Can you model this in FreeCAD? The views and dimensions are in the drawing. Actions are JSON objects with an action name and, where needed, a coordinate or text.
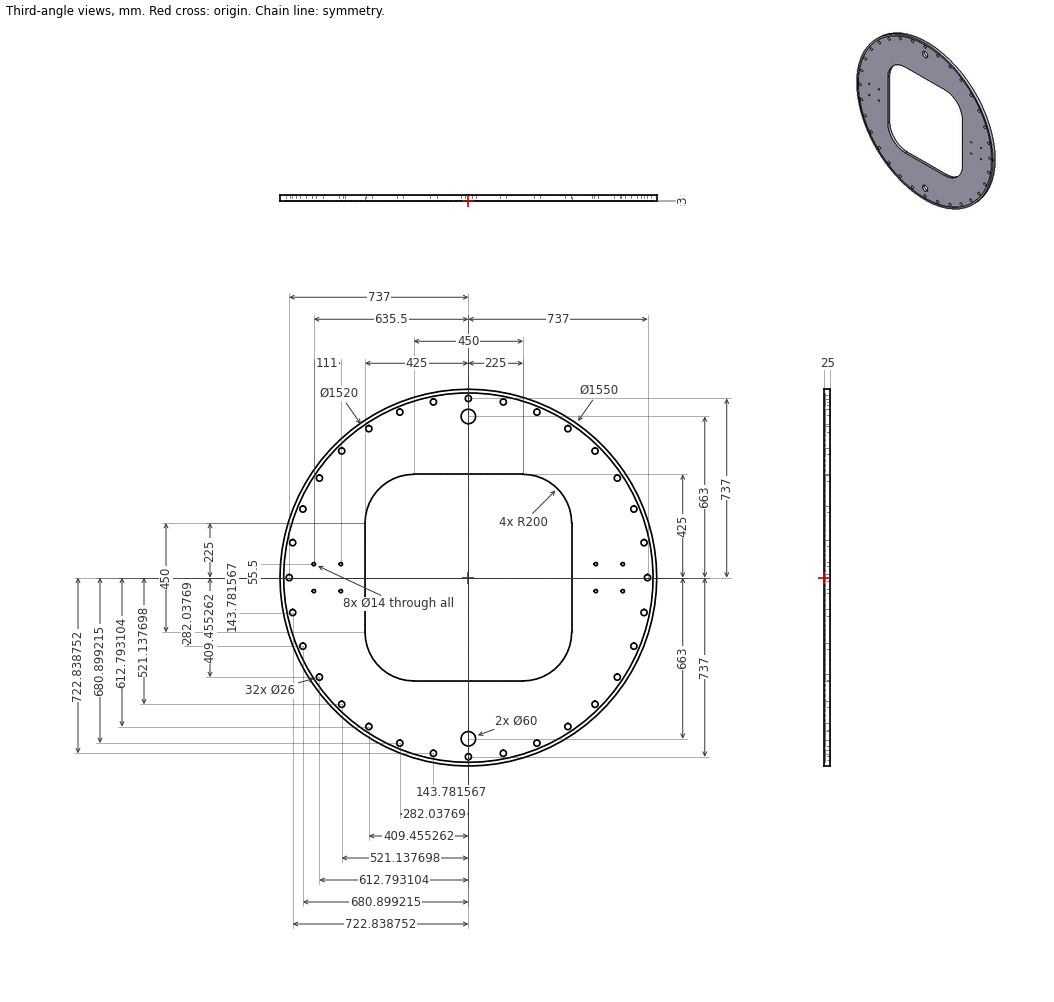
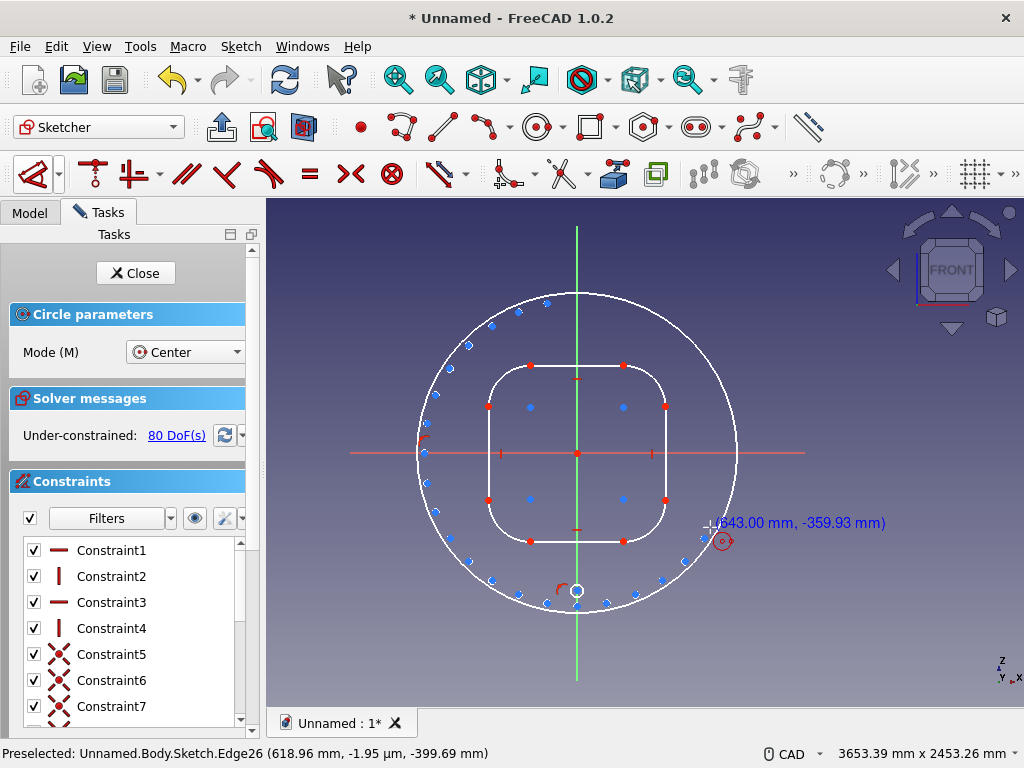
{"action": "scroll", "coordinate": [718, 512], "scroll_direction": "up", "scroll_amount": 4}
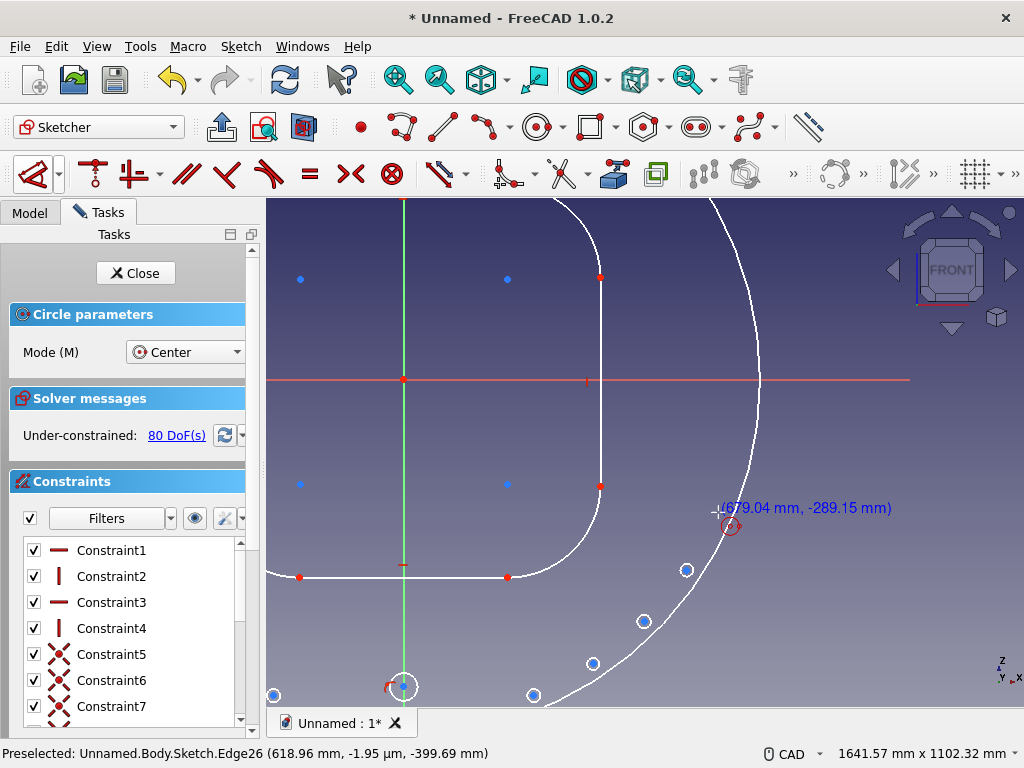
{"action": "left_click", "coordinate": [718, 510]}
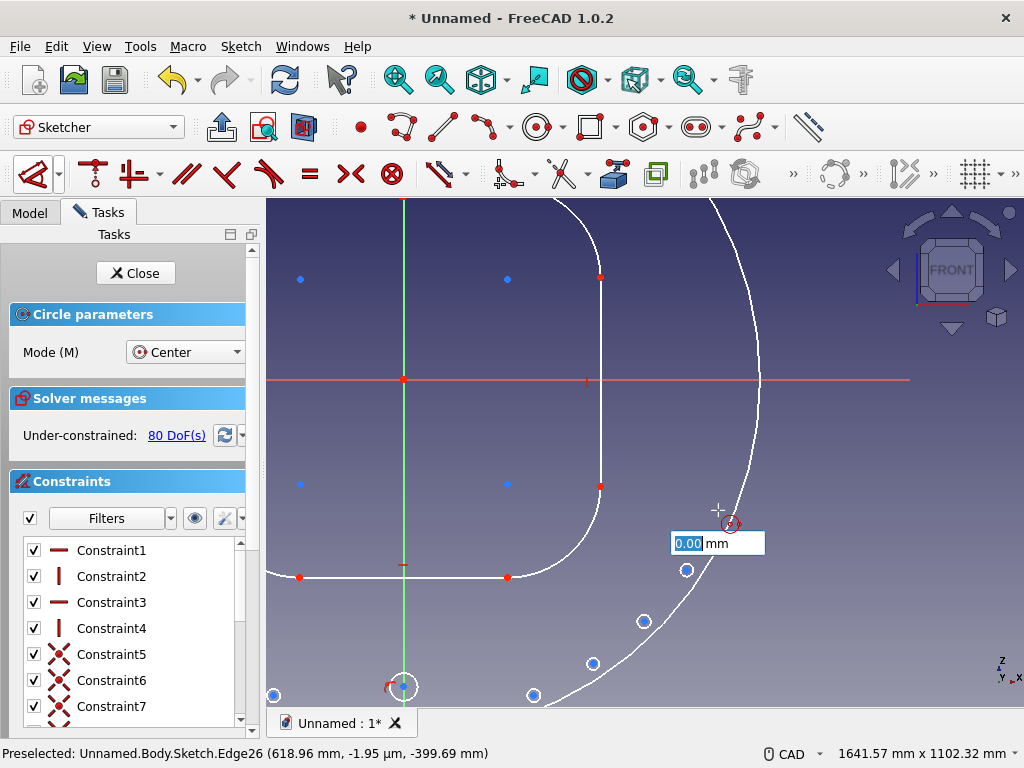
{"action": "scroll", "coordinate": [722, 506], "scroll_direction": "up", "scroll_amount": 5}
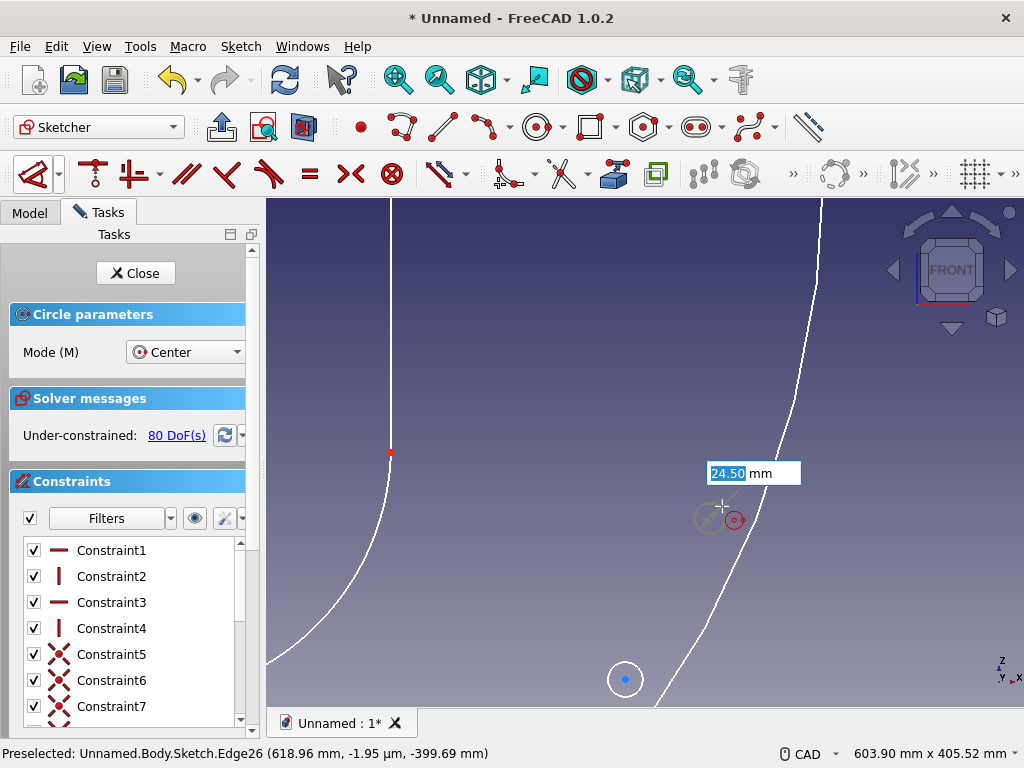
{"action": "left_click", "coordinate": [722, 505]}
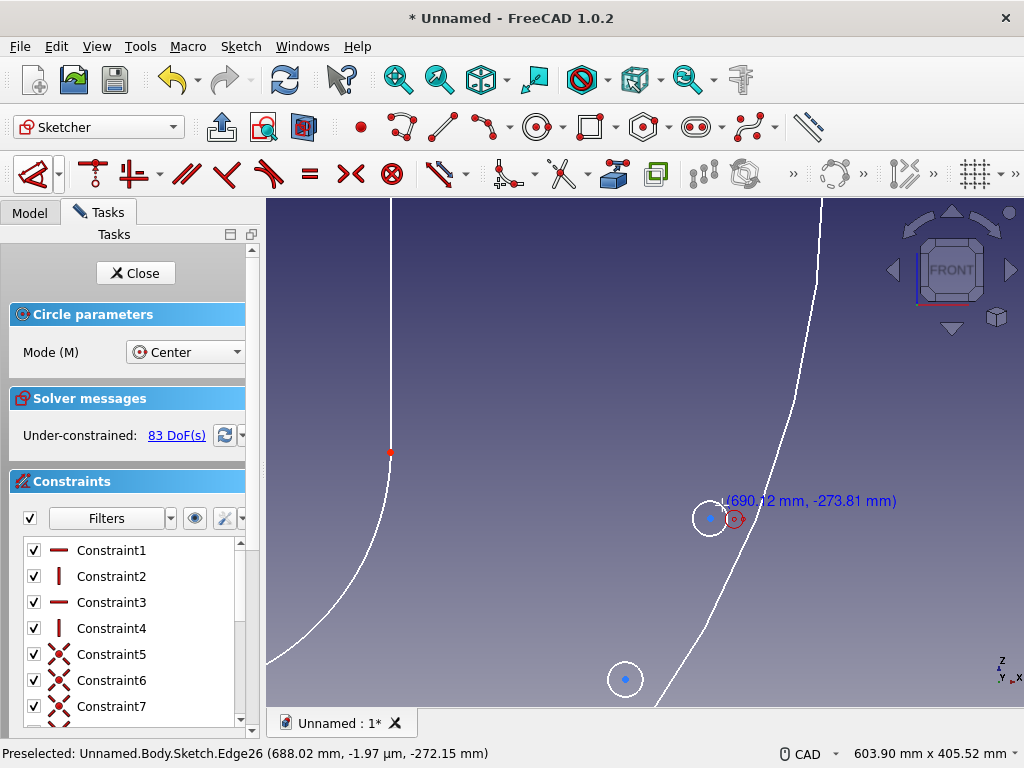
{"action": "scroll", "coordinate": [763, 343], "scroll_direction": "up", "scroll_amount": 2}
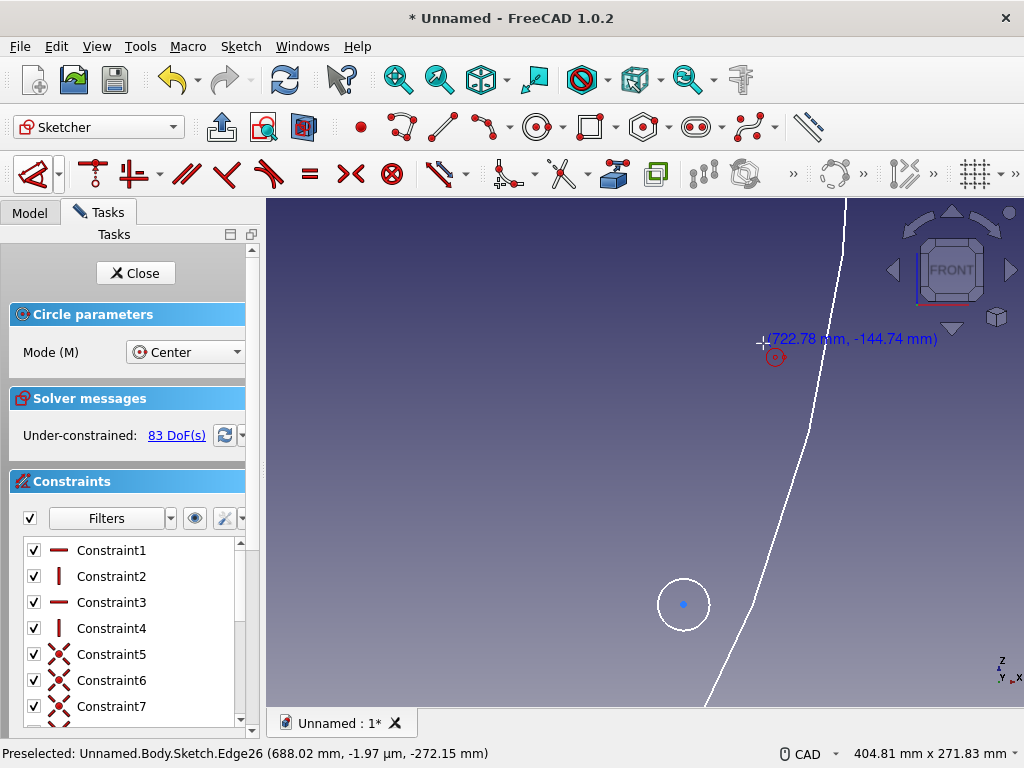
{"action": "scroll", "coordinate": [722, 500], "scroll_direction": "down", "scroll_amount": 11}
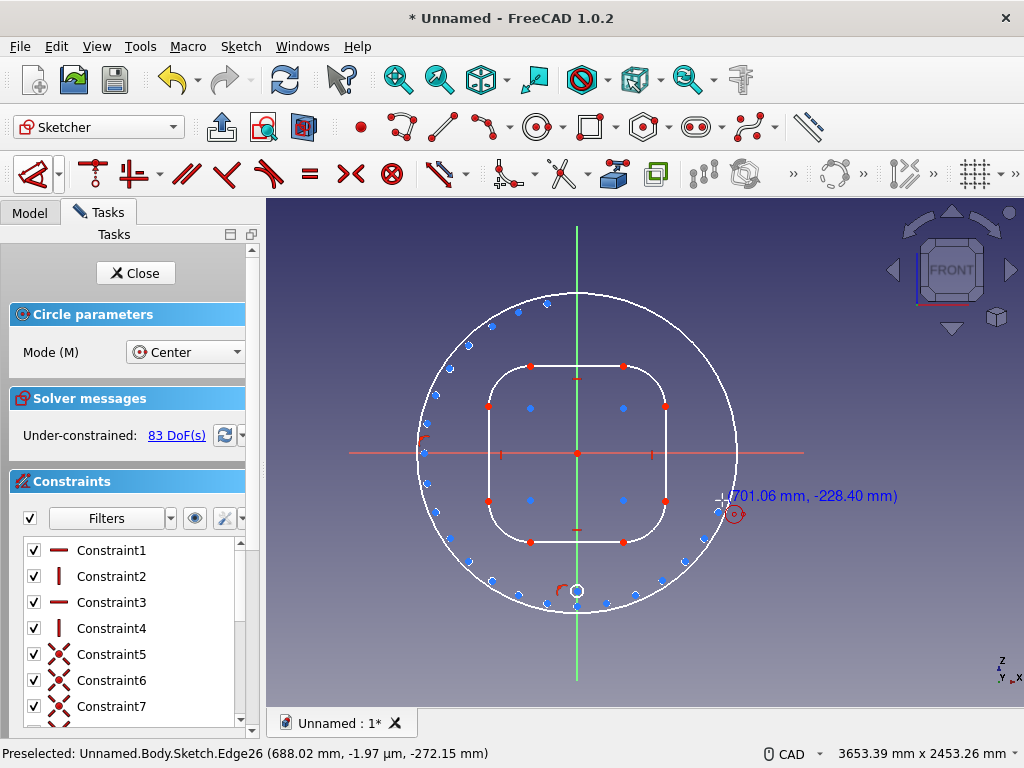
{"action": "scroll", "coordinate": [727, 483], "scroll_direction": "up", "scroll_amount": 4}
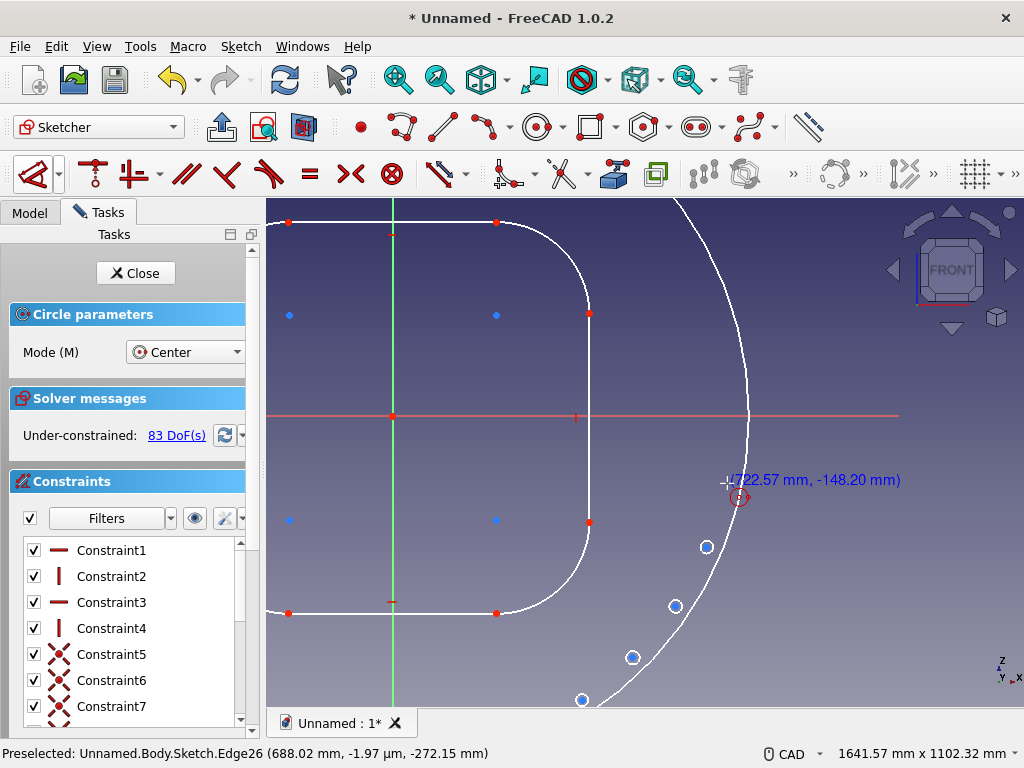
{"action": "left_click", "coordinate": [726, 482]}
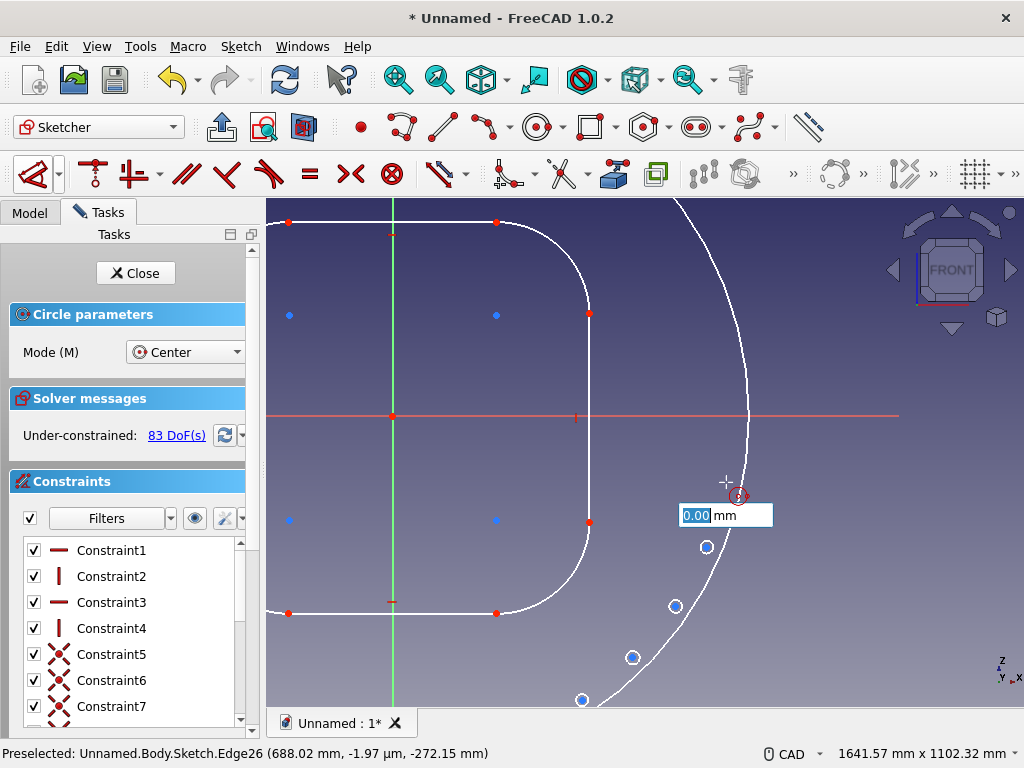
{"action": "scroll", "coordinate": [731, 478], "scroll_direction": "up", "scroll_amount": 5}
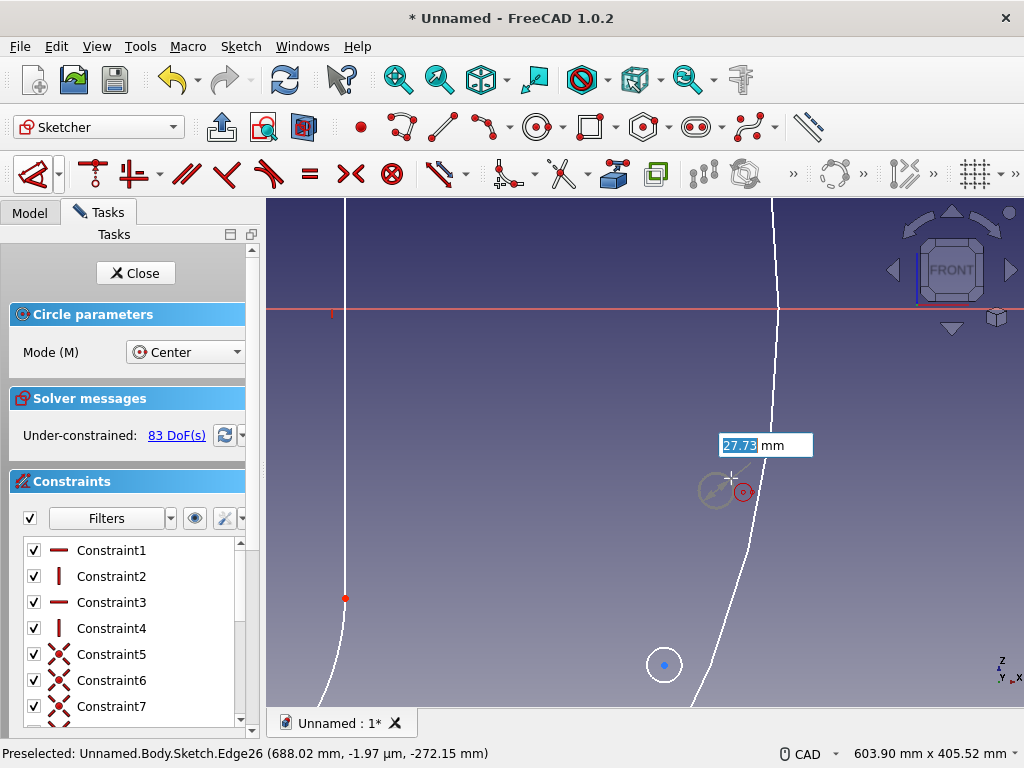
{"action": "left_click", "coordinate": [729, 478]}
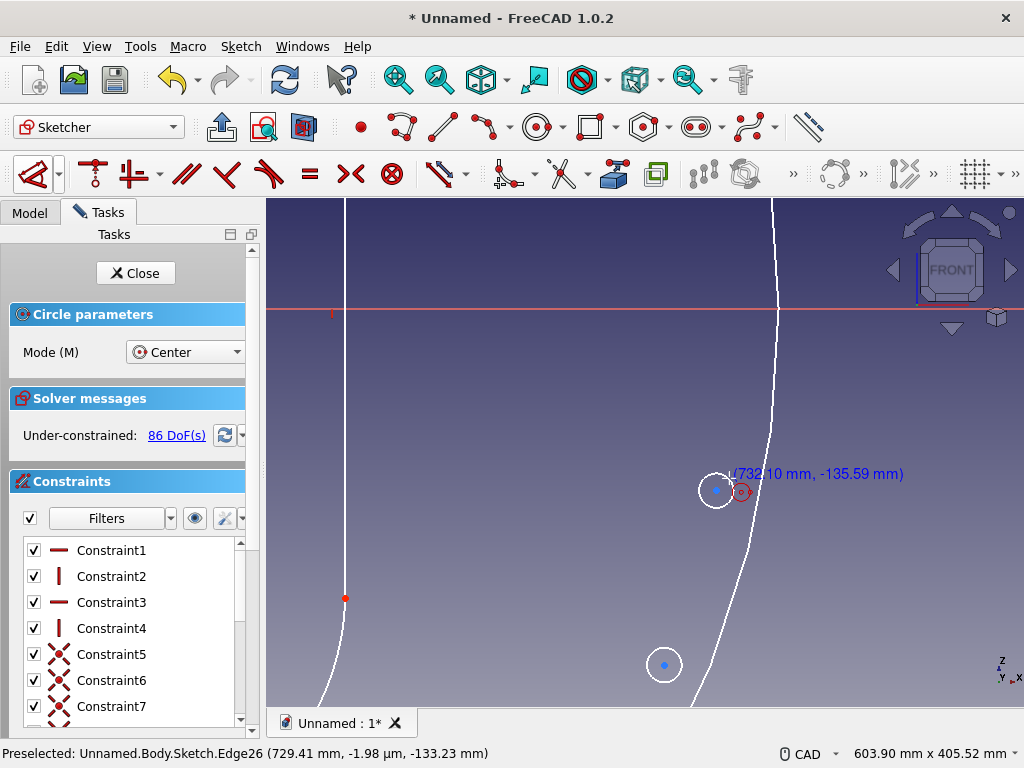
{"action": "scroll", "coordinate": [735, 309], "scroll_direction": "up", "scroll_amount": 2}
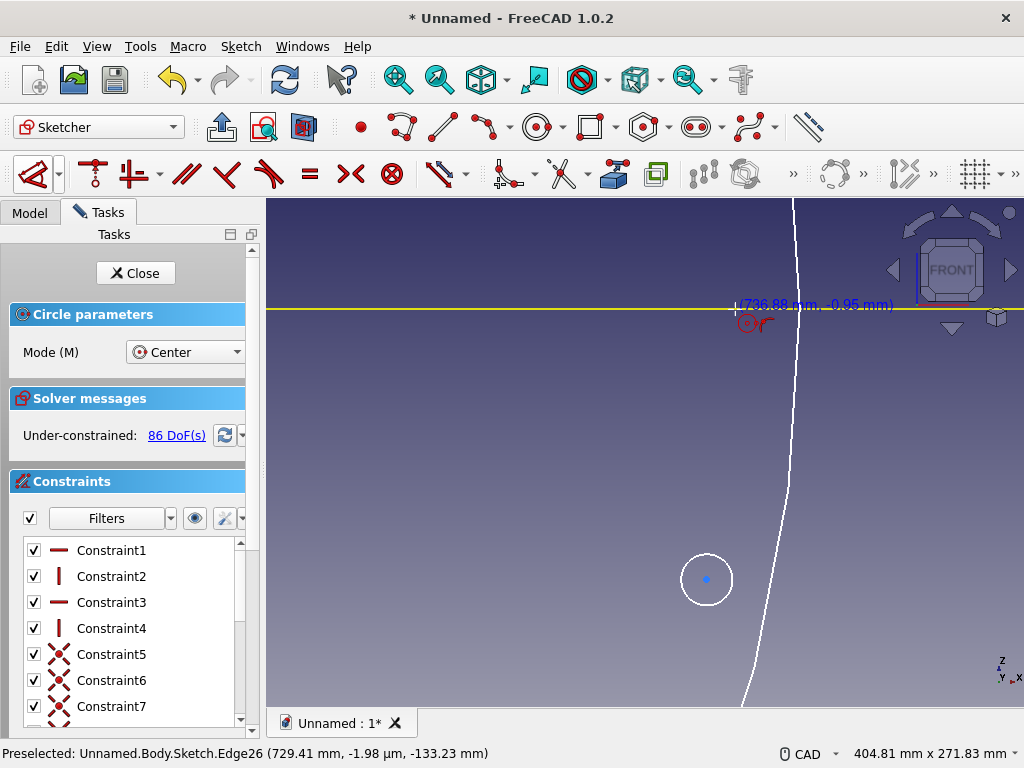
{"action": "scroll", "coordinate": [729, 470], "scroll_direction": "down", "scroll_amount": 11}